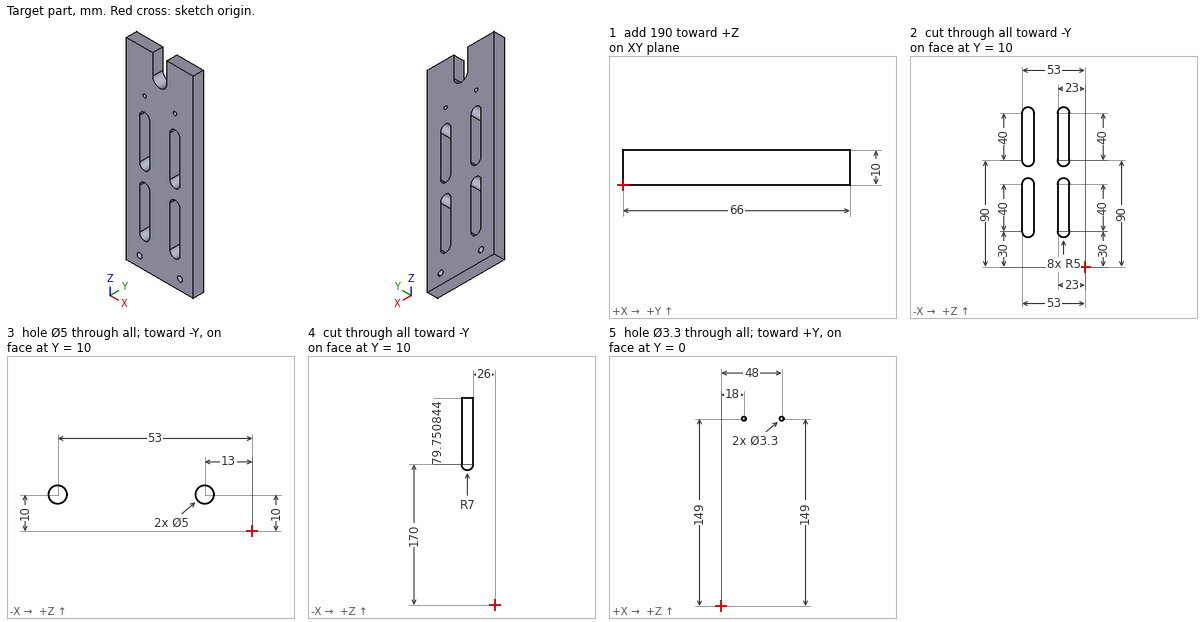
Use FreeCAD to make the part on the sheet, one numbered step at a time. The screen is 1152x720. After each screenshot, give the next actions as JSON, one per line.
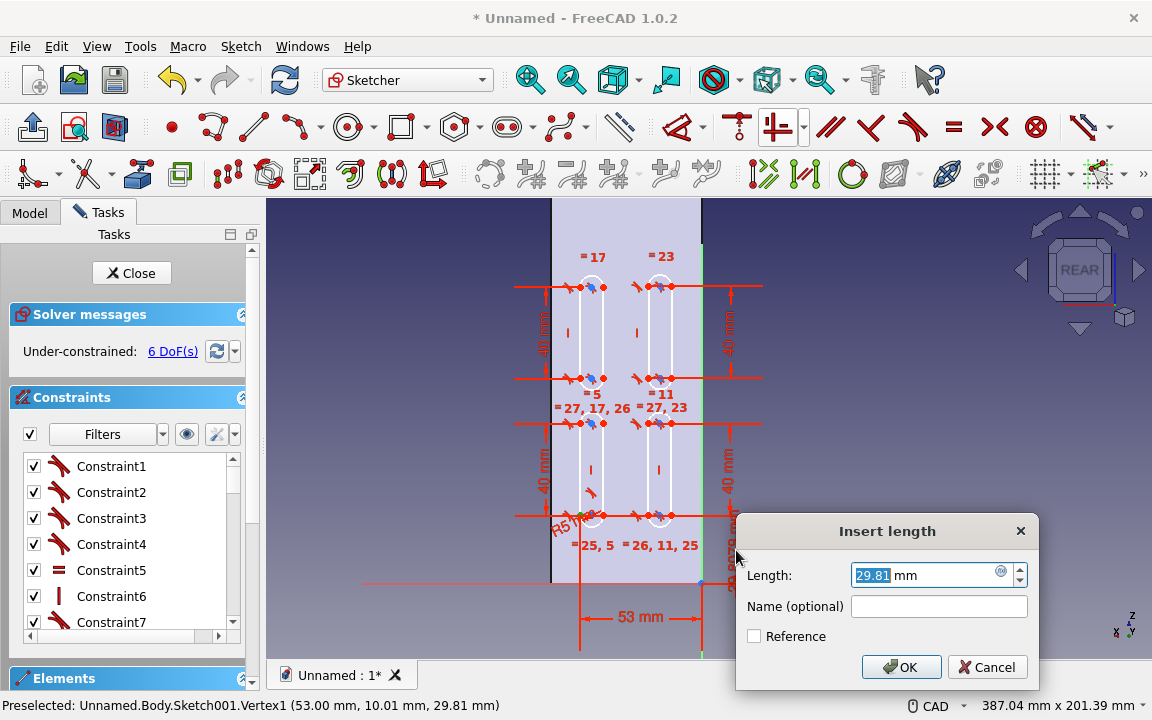
{"action": "type", "text": "30"}
{"action": "key", "text": "Return"}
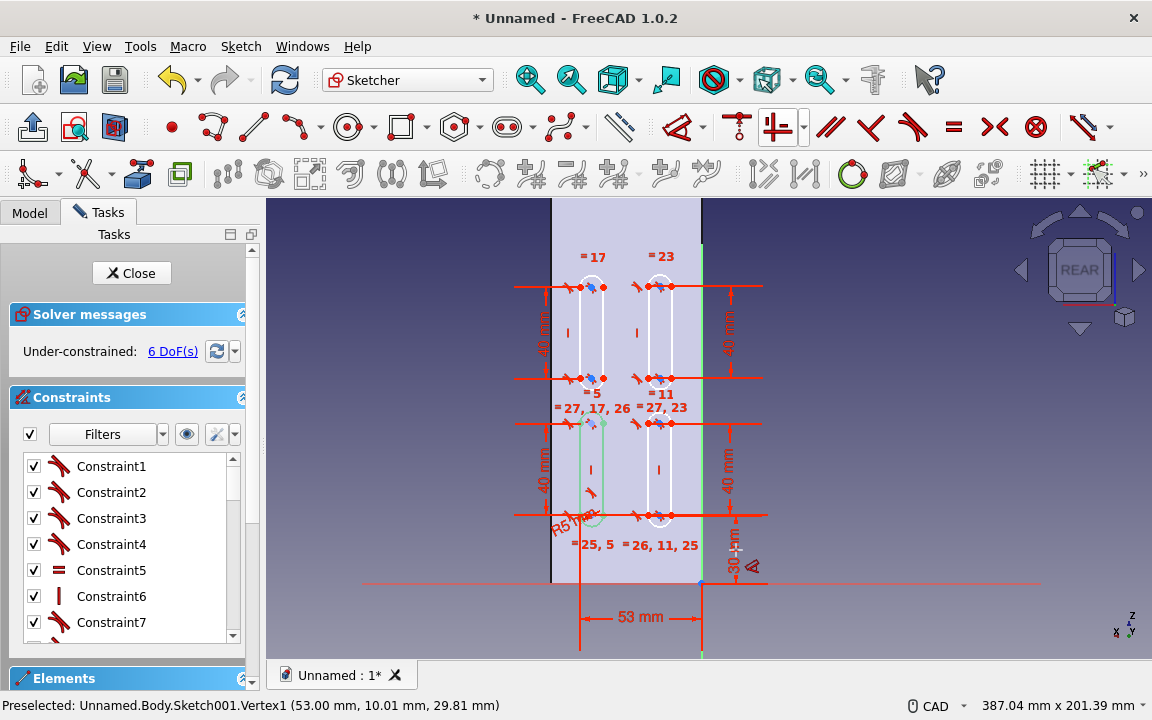
{"action": "left_click", "coordinate": [648, 516]}
{"action": "left_click", "coordinate": [687, 434]}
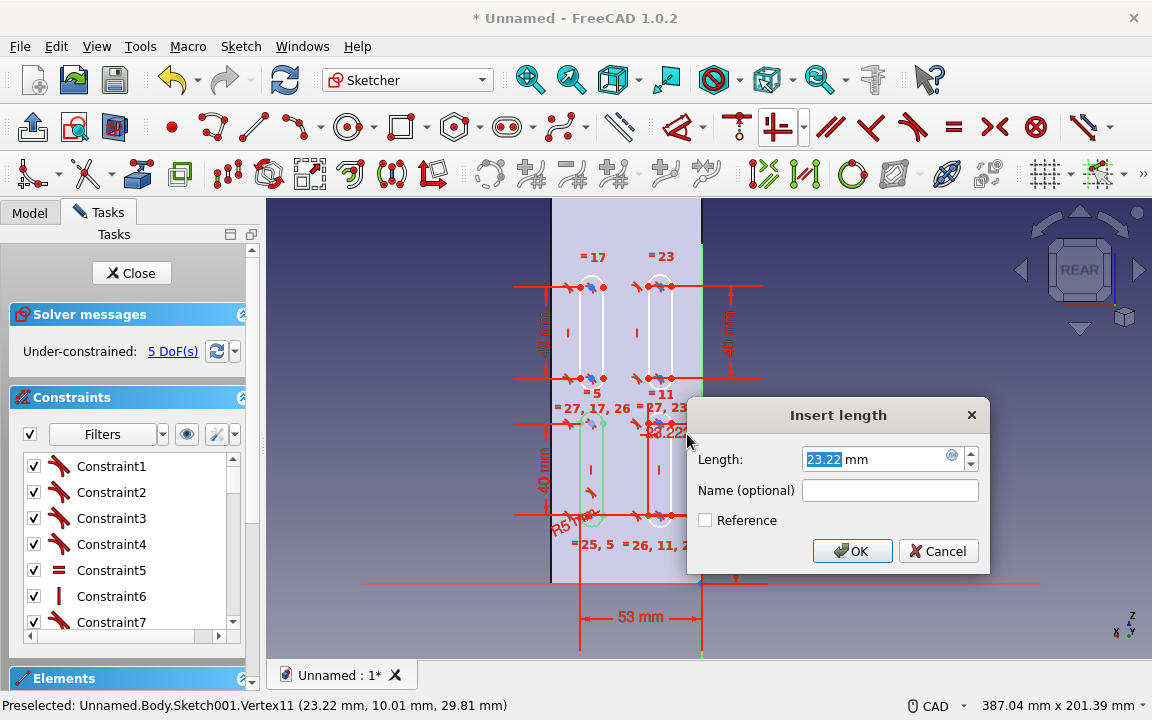
{"action": "type", "text": "23"}
{"action": "key", "text": "Return"}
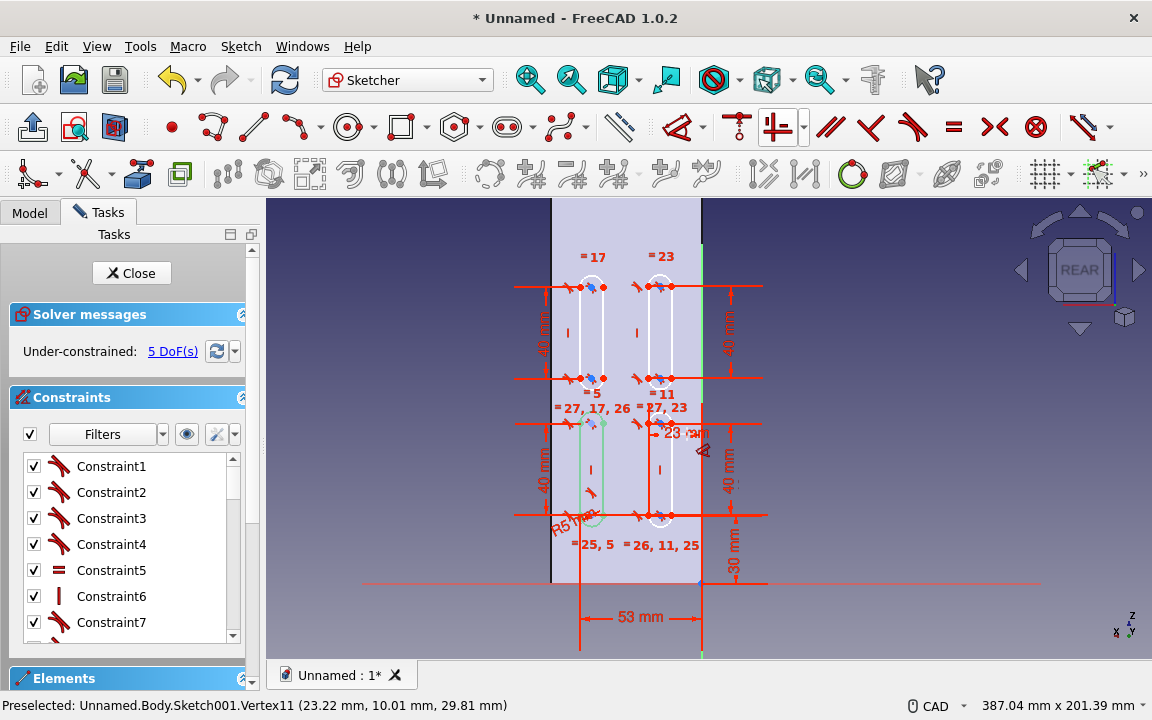
{"action": "left_click", "coordinate": [649, 516]}
{"action": "left_click", "coordinate": [736, 526]}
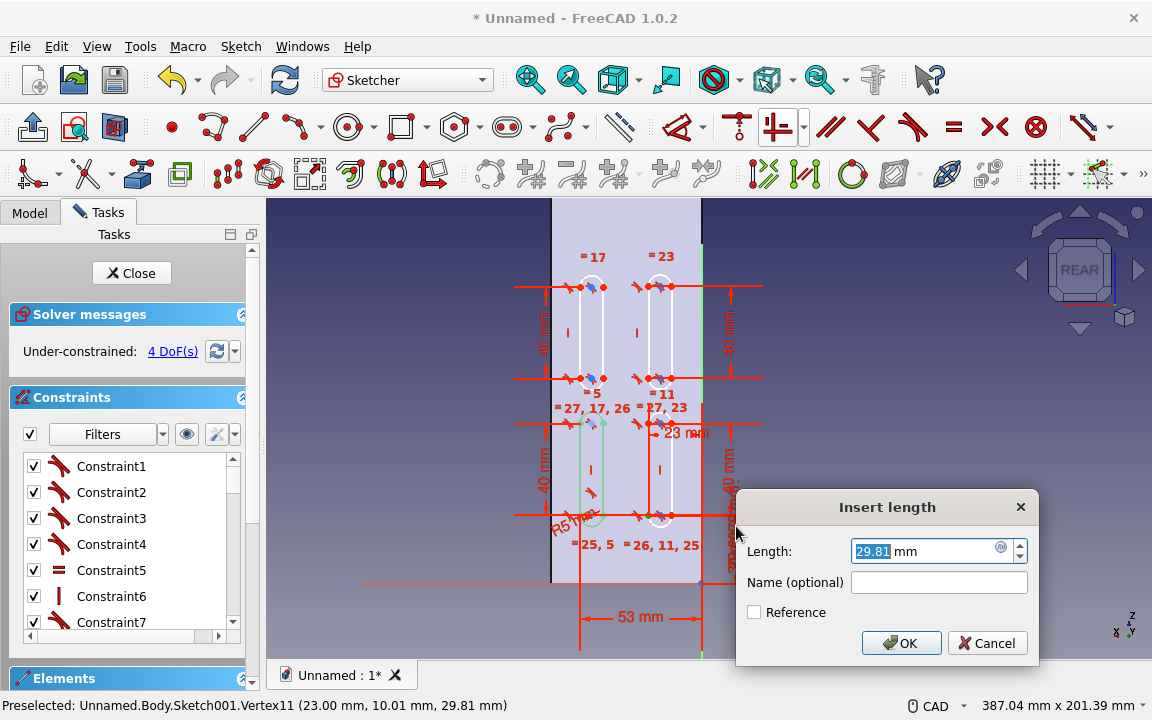
{"action": "type", "text": "30"}
{"action": "key", "text": "Return"}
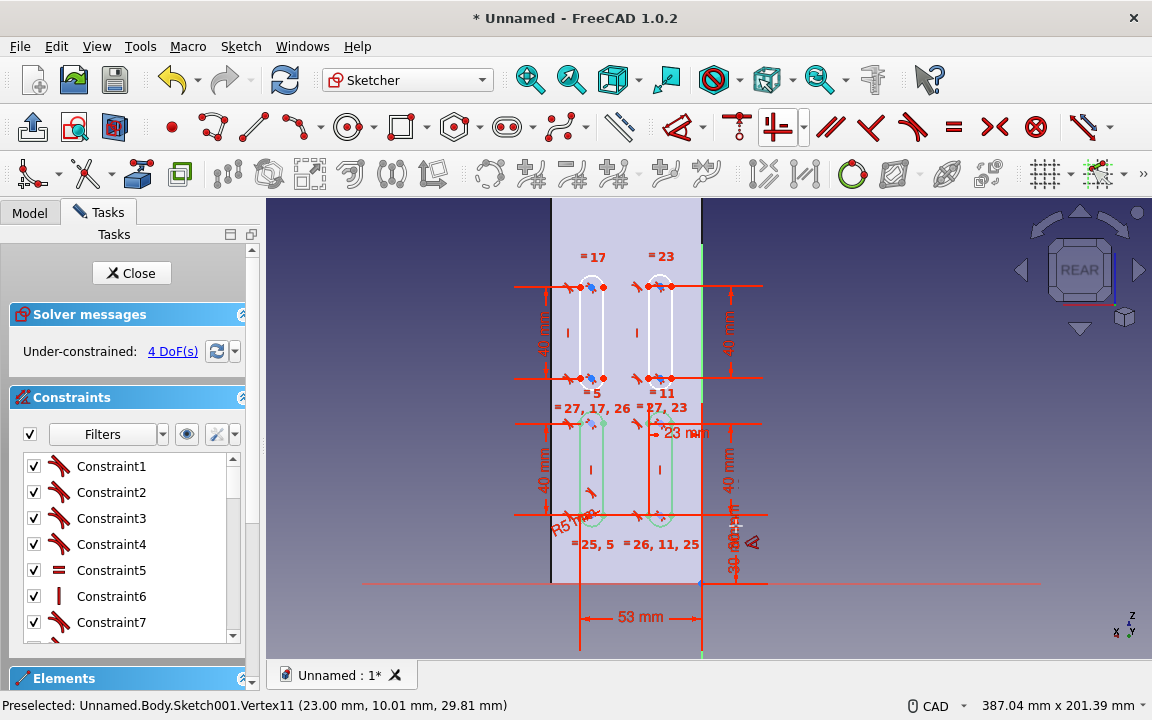
{"action": "left_click", "coordinate": [580, 379]}
{"action": "left_click", "coordinate": [613, 273]}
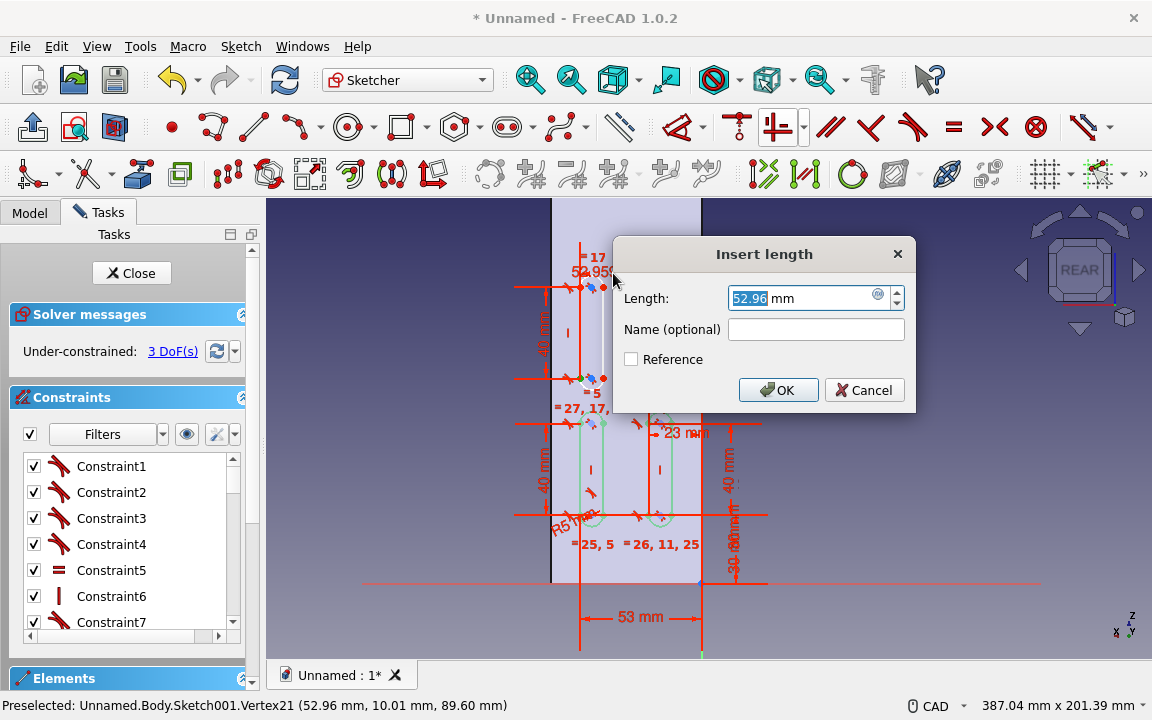
{"action": "type", "text": "53"}
{"action": "key", "text": "Return"}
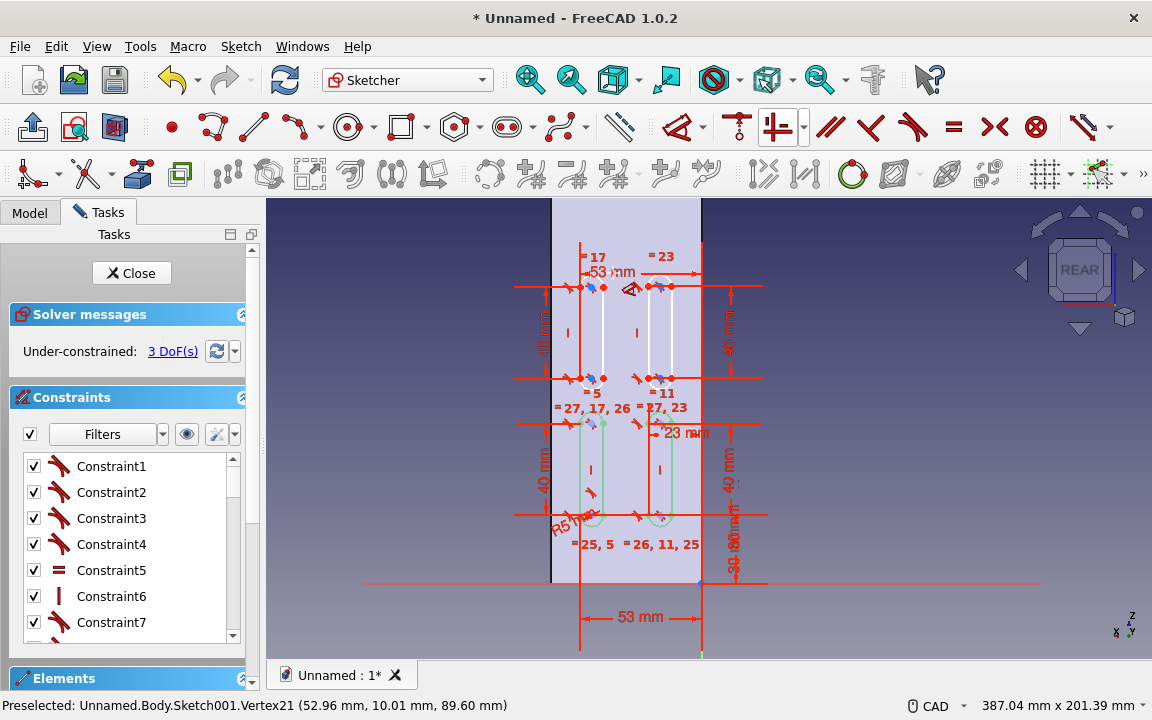
{"action": "left_click", "coordinate": [580, 379]}
{"action": "left_click", "coordinate": [736, 409]}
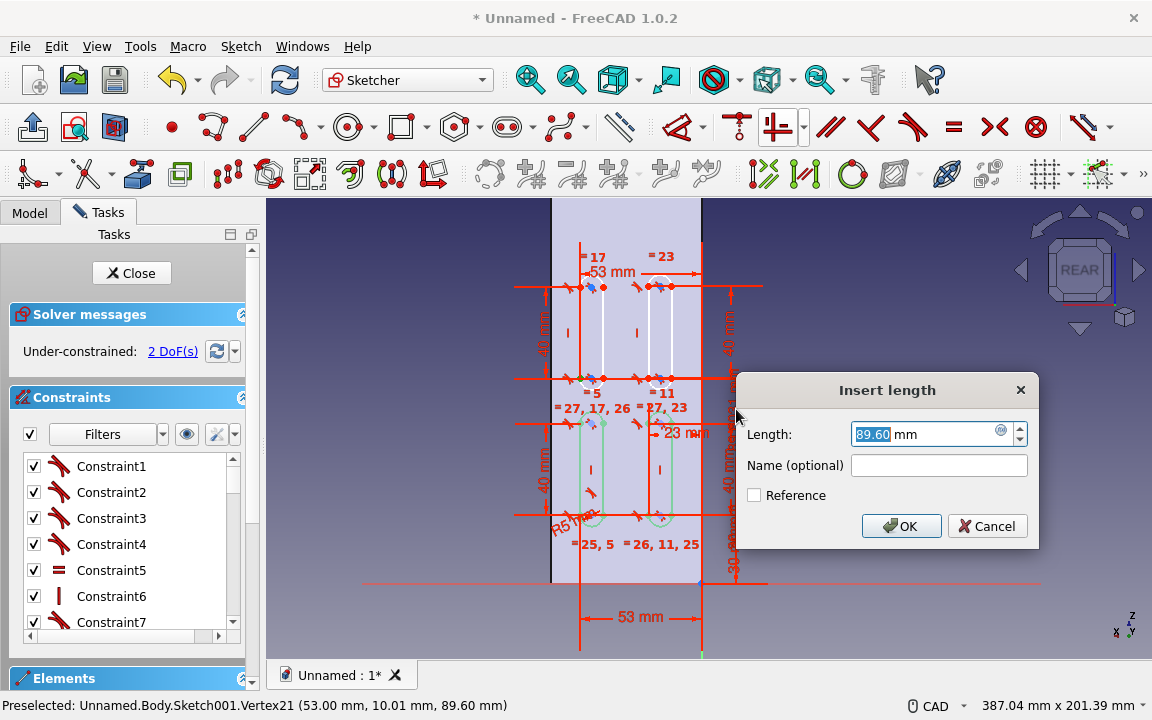
{"action": "type", "text": "90"}
{"action": "key", "text": "Return"}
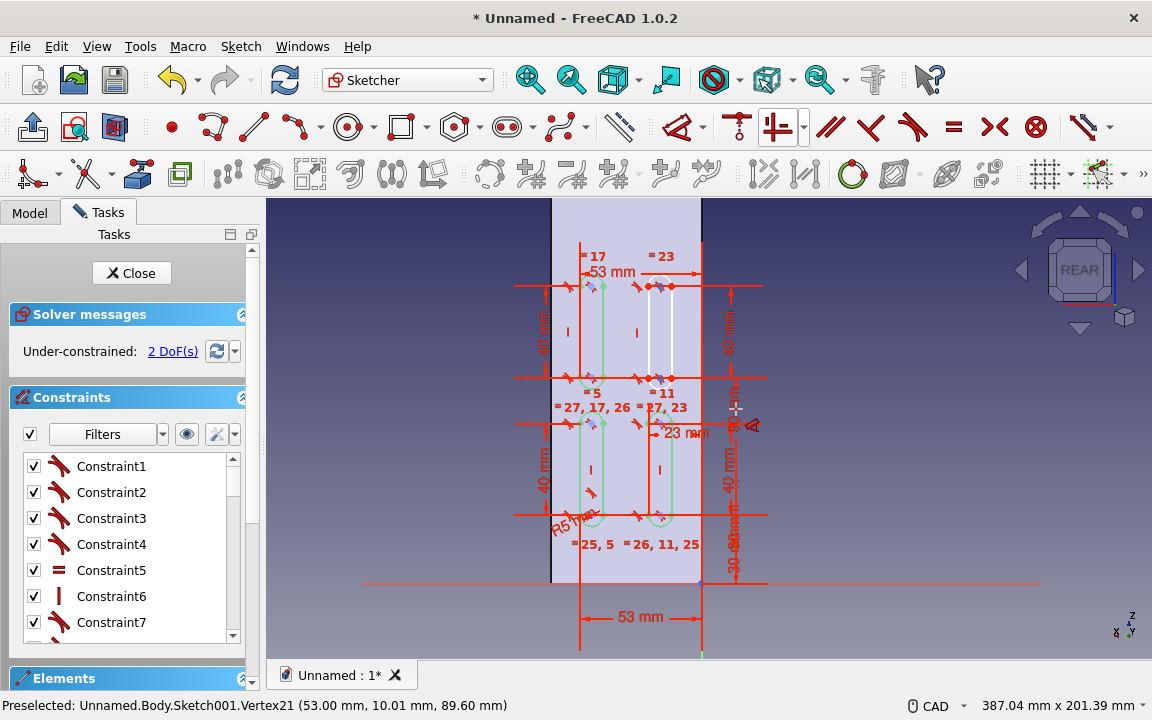
{"action": "left_click", "coordinate": [649, 378]}
{"action": "left_click", "coordinate": [687, 296]}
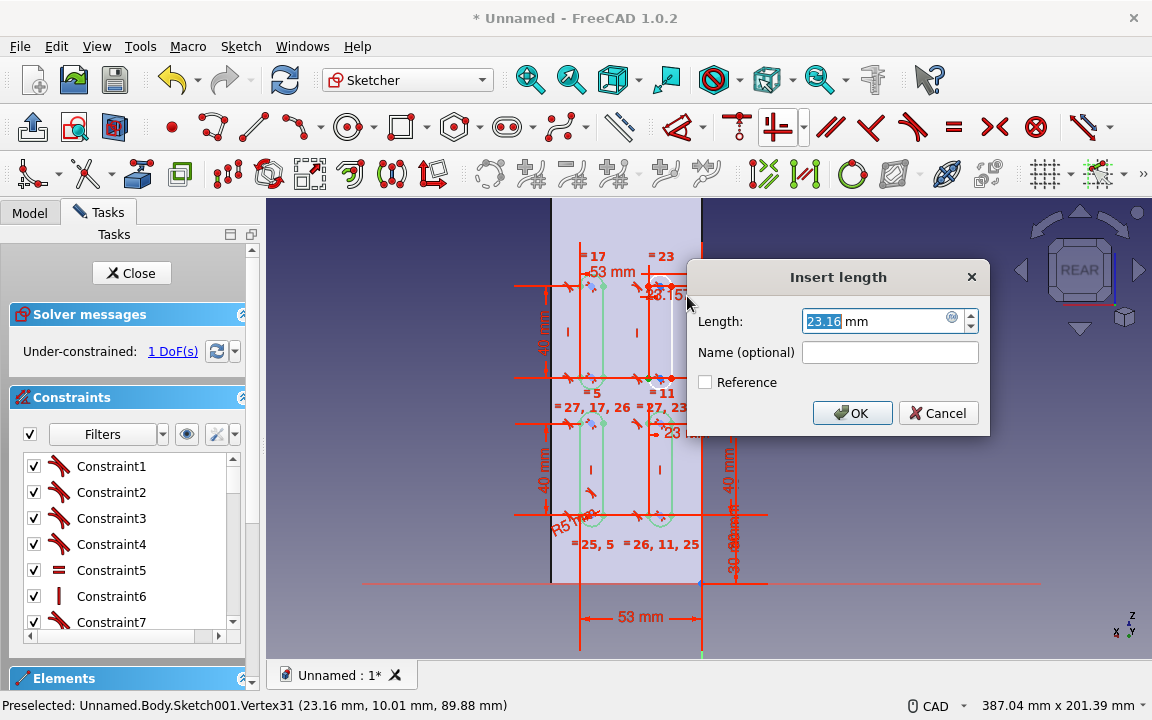
{"action": "type", "text": "23"}
{"action": "key", "text": "Return"}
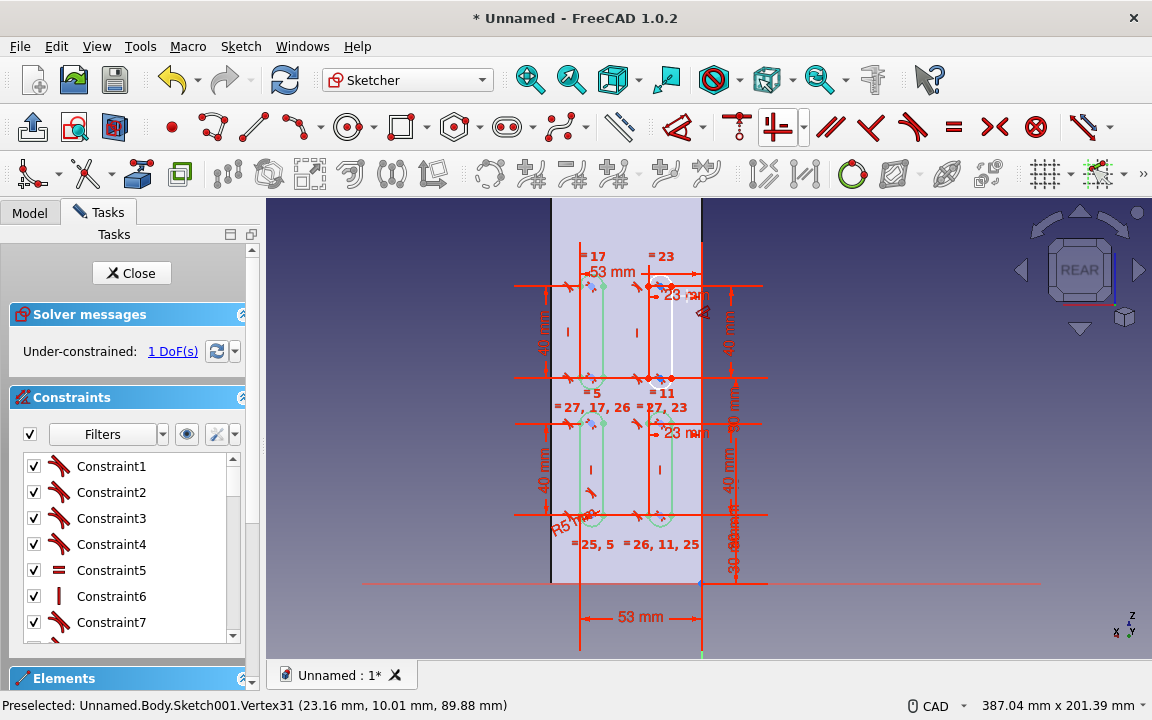
{"action": "left_click", "coordinate": [649, 378]}
{"action": "left_click", "coordinate": [615, 409]}